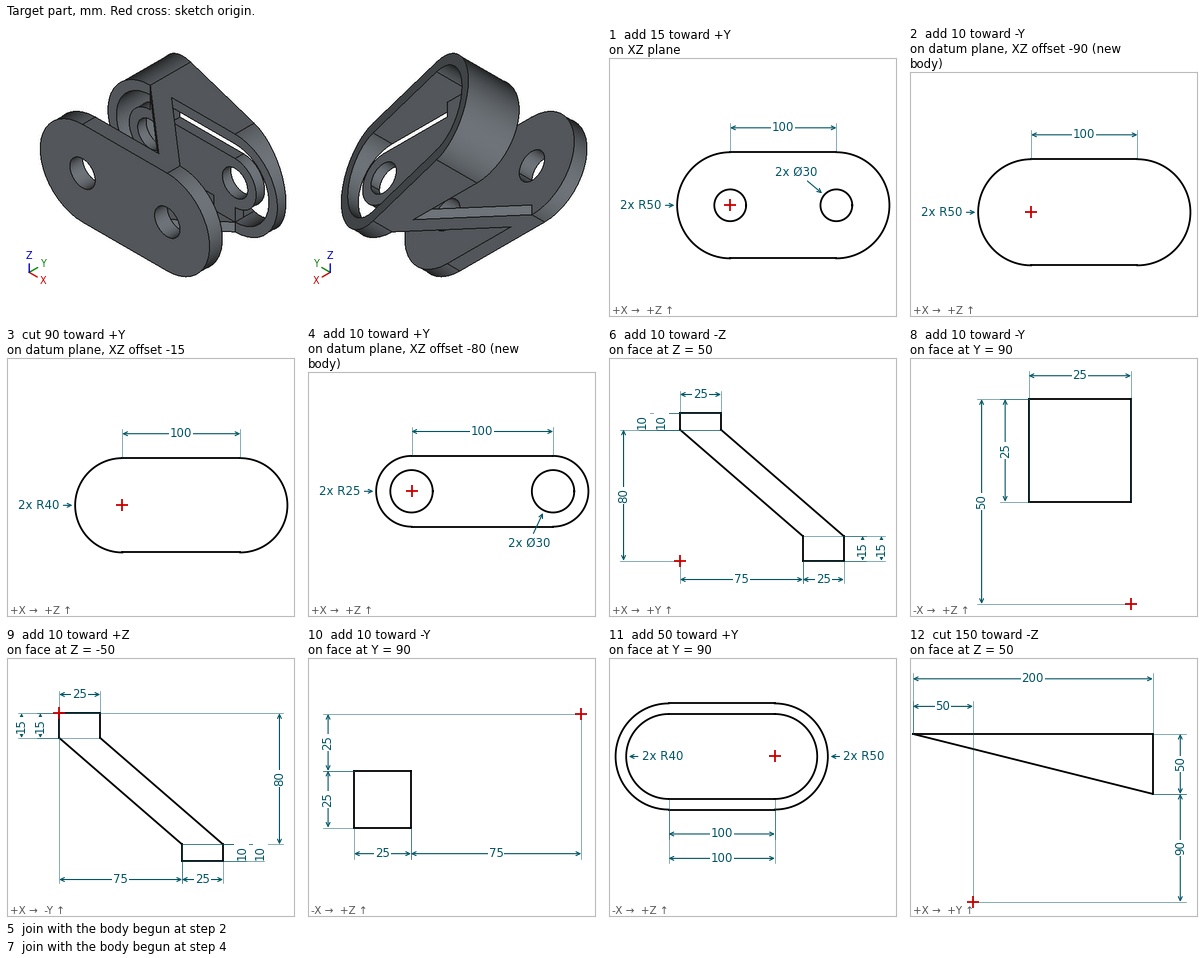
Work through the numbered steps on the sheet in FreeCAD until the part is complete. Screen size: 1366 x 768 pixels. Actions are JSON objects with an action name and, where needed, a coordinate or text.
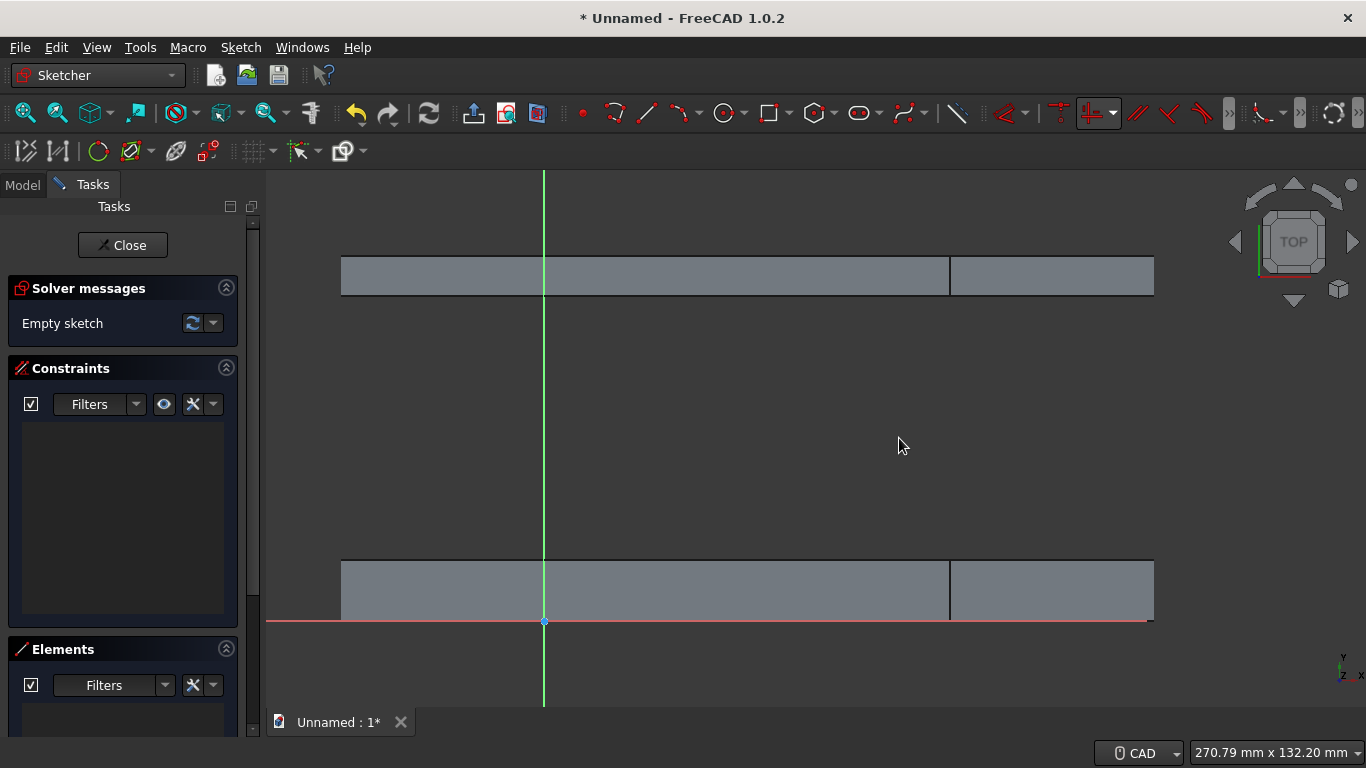
{"action": "left_click", "coordinate": [616, 114]}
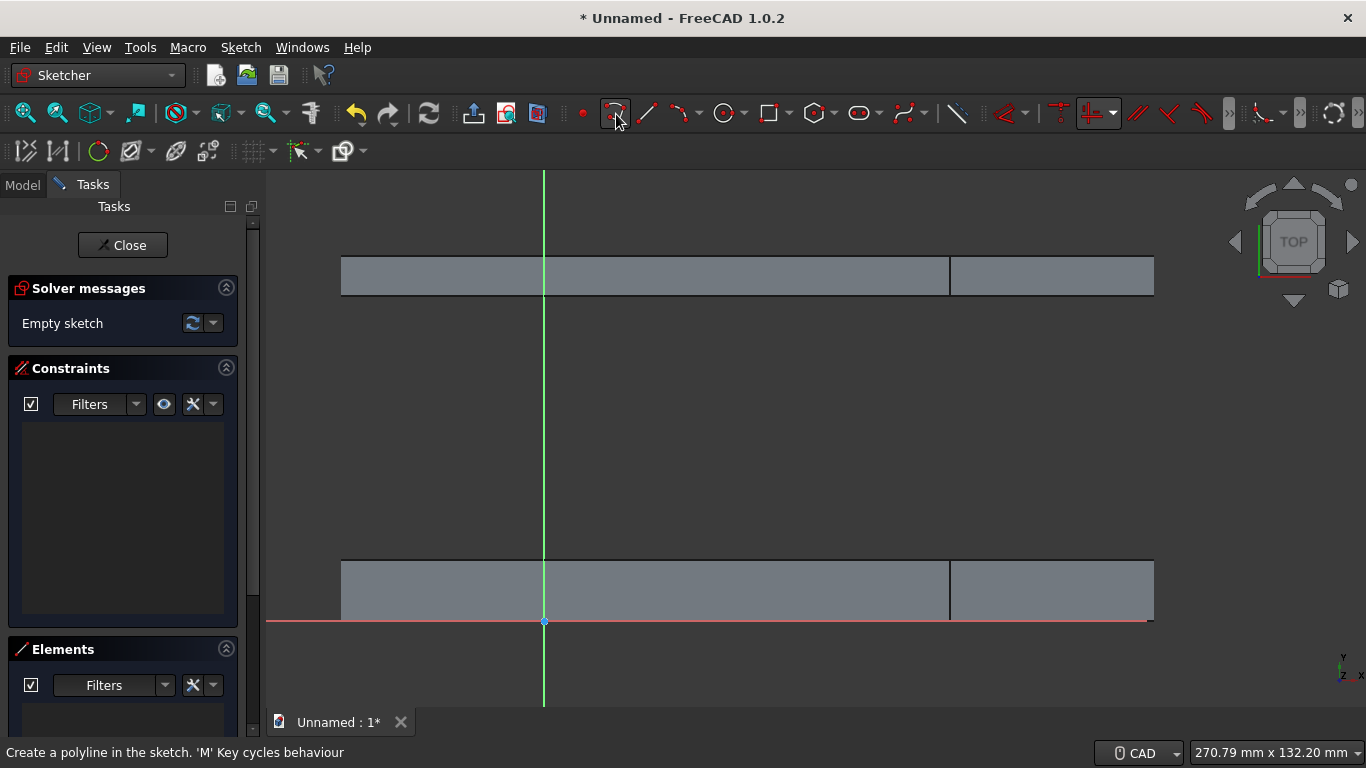
{"action": "left_click", "coordinate": [849, 621]}
{"action": "left_click", "coordinate": [950, 612]}
{"action": "left_click", "coordinate": [950, 560]}
{"action": "left_click", "coordinate": [646, 296]}
{"action": "left_click", "coordinate": [646, 256]}
{"action": "left_click", "coordinate": [544, 256]}
{"action": "left_click", "coordinate": [553, 296]}
{"action": "left_click", "coordinate": [849, 560]}
{"action": "left_click", "coordinate": [849, 621]}
{"action": "key", "text": "Escape"}
{"action": "key", "text": "Escape"}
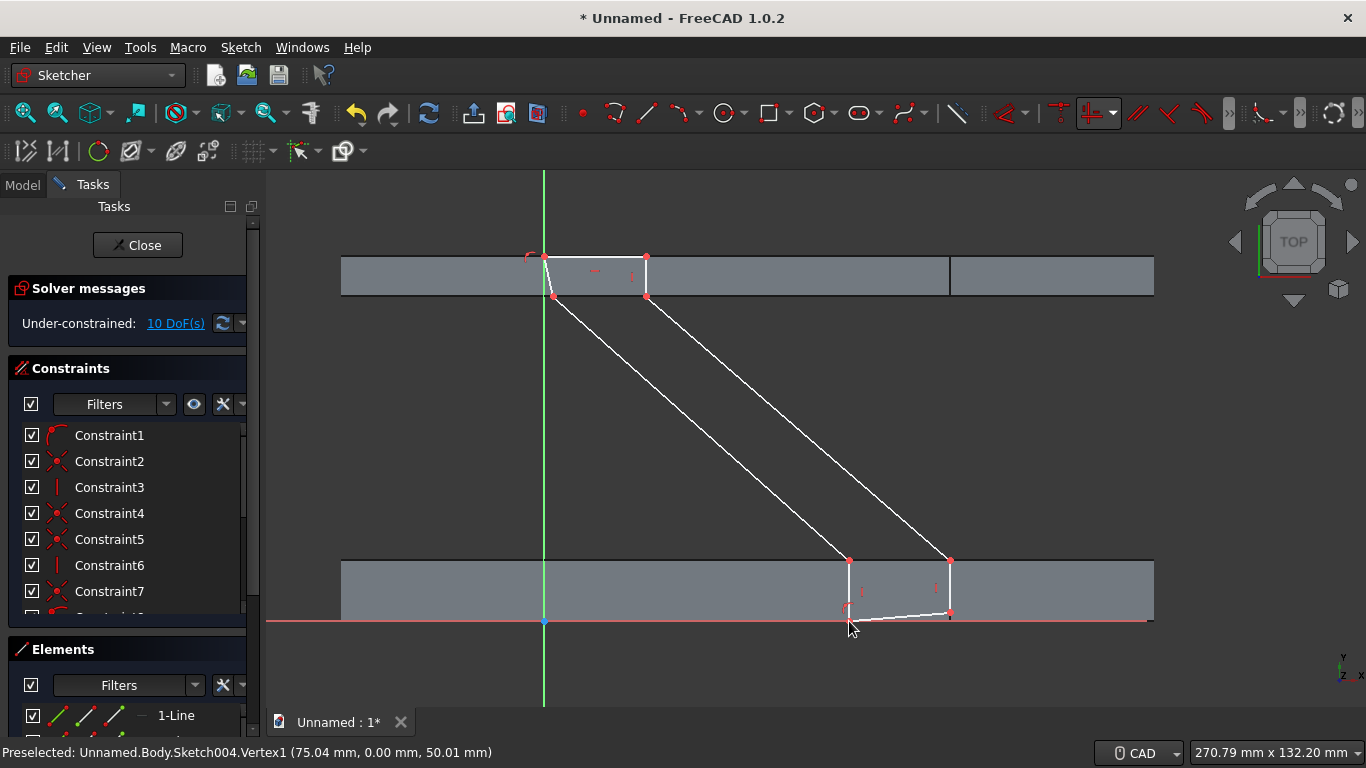
{"action": "left_click", "coordinate": [879, 619]}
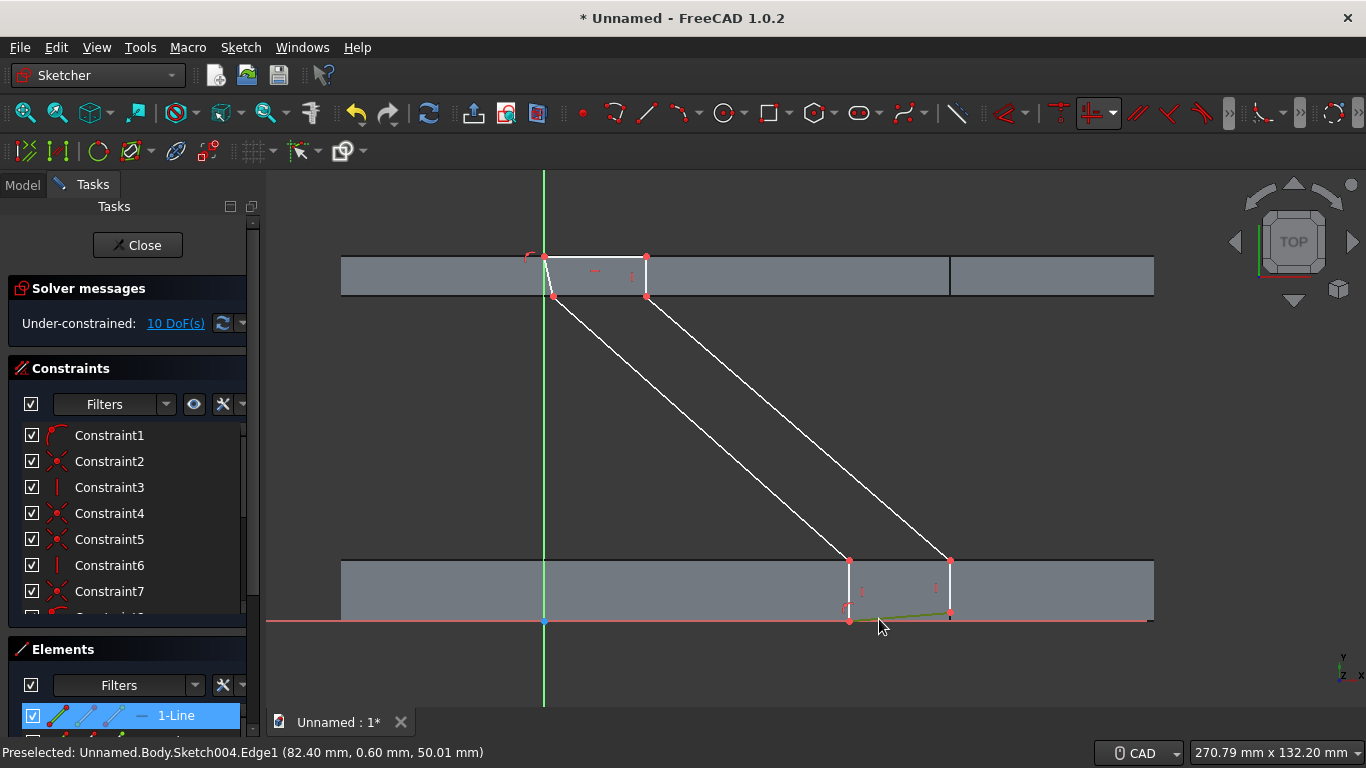
{"action": "left_click", "coordinate": [1116, 114]}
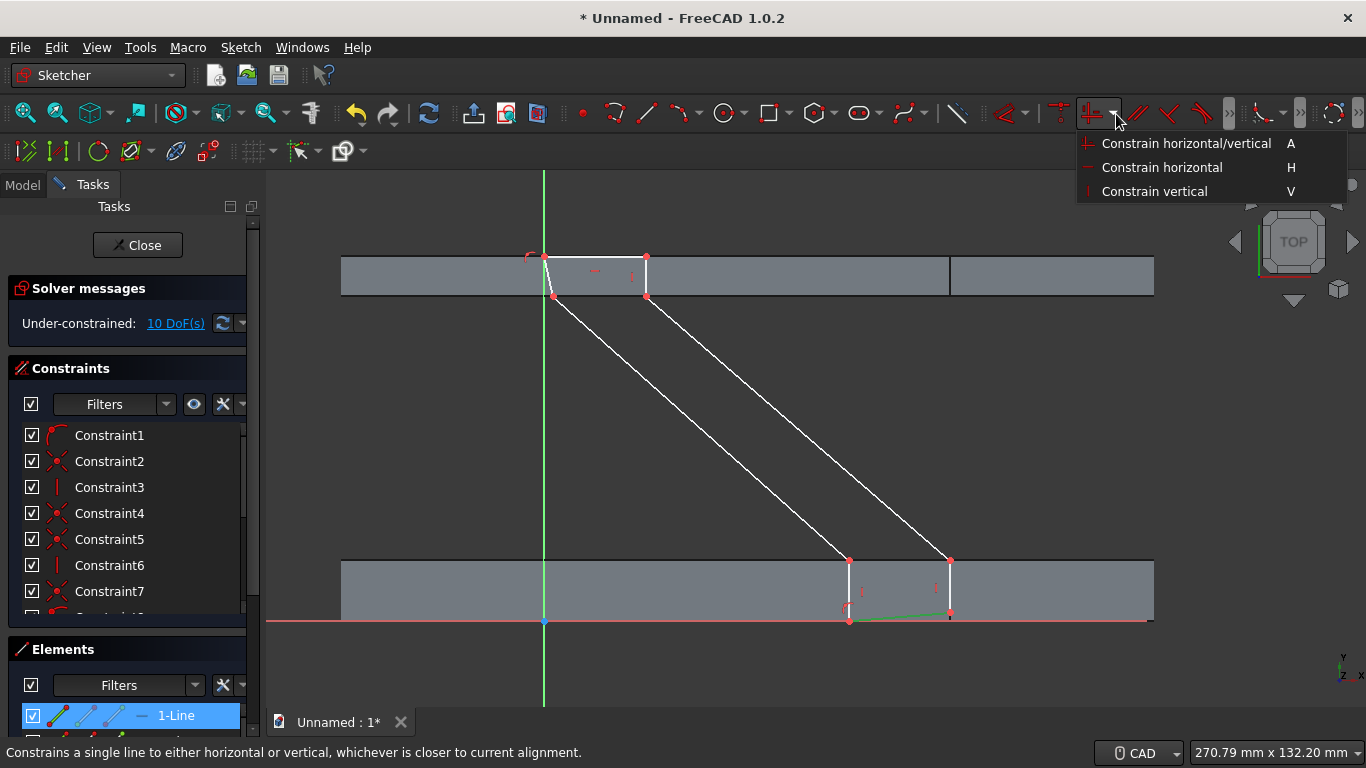
{"action": "left_click", "coordinate": [1212, 167]}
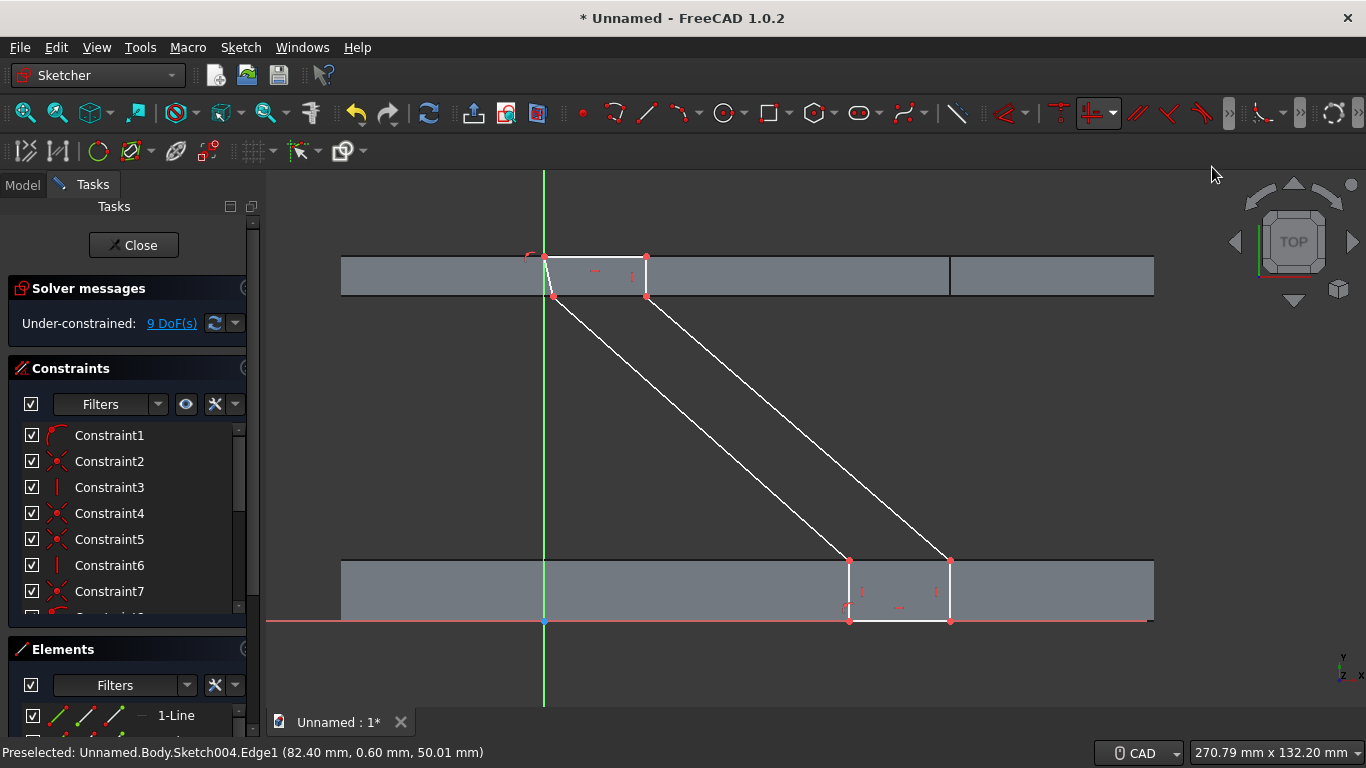
{"action": "left_click", "coordinate": [547, 269]}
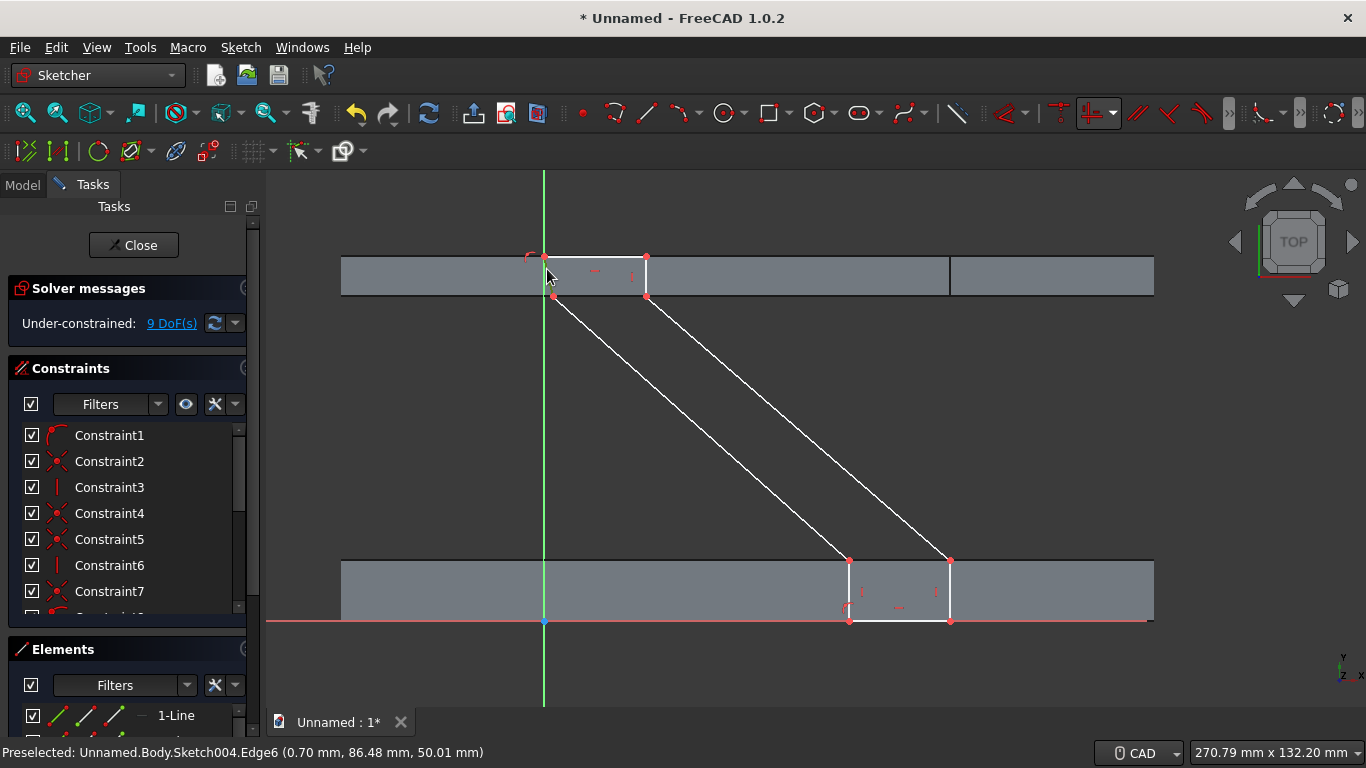
{"action": "key", "text": "v"}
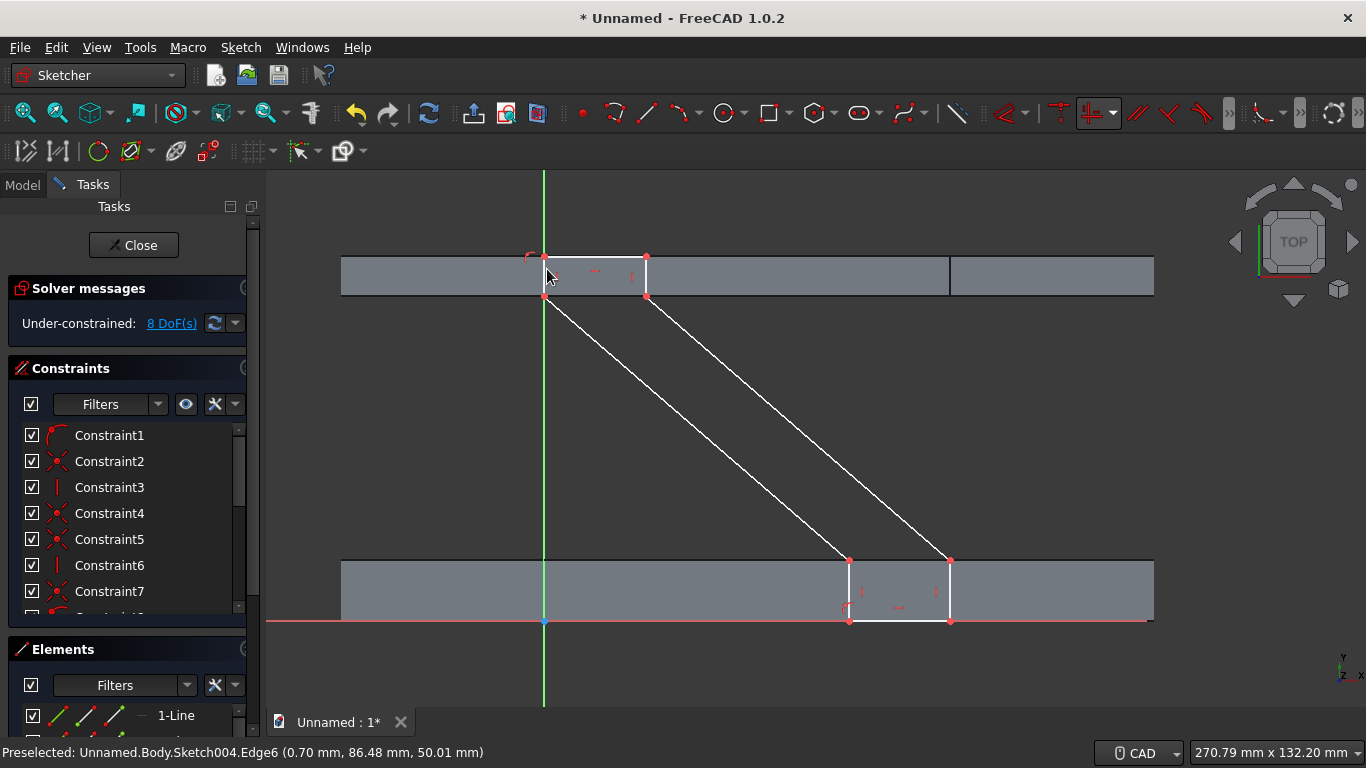
{"action": "left_click", "coordinate": [1004, 114]}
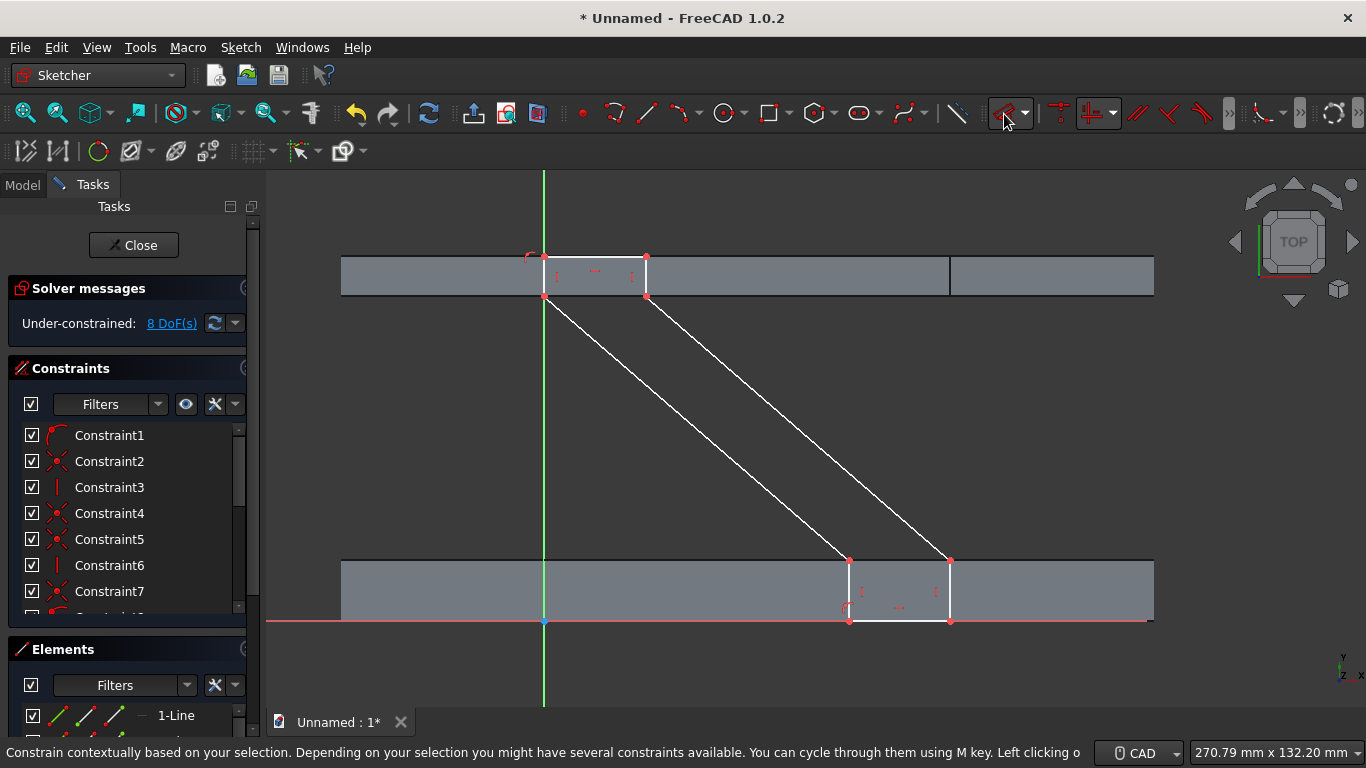
{"action": "left_click", "coordinate": [879, 621]}
{"action": "left_click", "coordinate": [899, 655]}